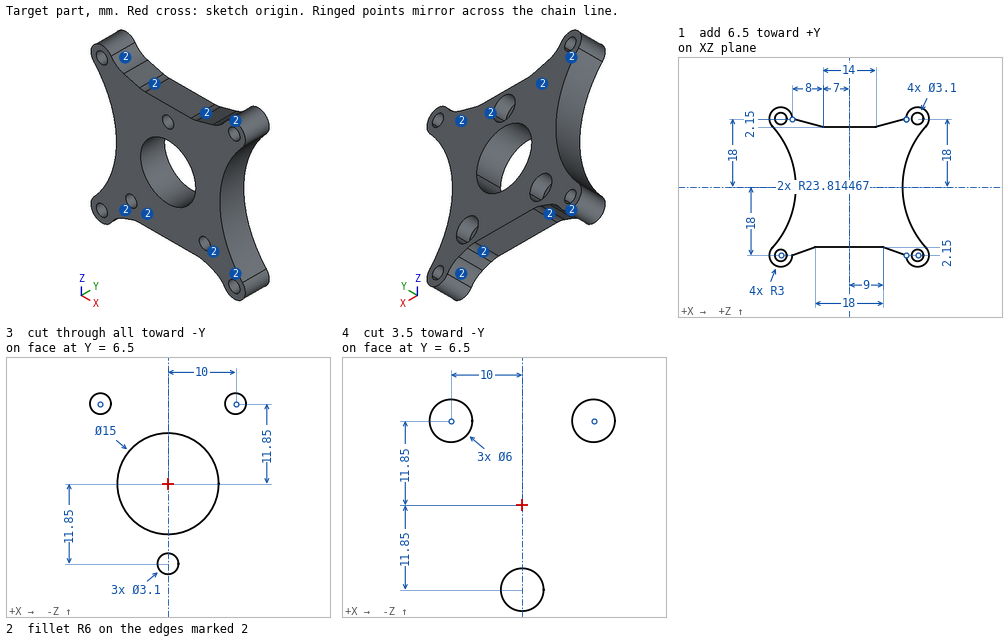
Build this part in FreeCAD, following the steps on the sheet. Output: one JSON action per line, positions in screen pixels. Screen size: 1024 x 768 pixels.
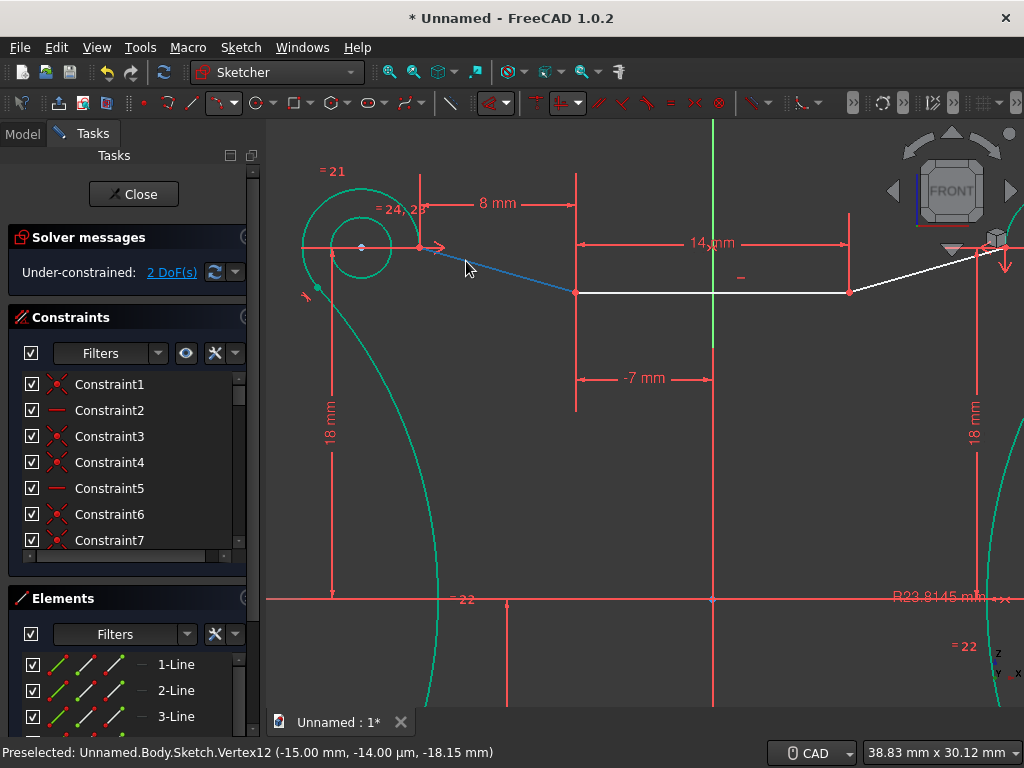
{"action": "left_click", "coordinate": [467, 261]}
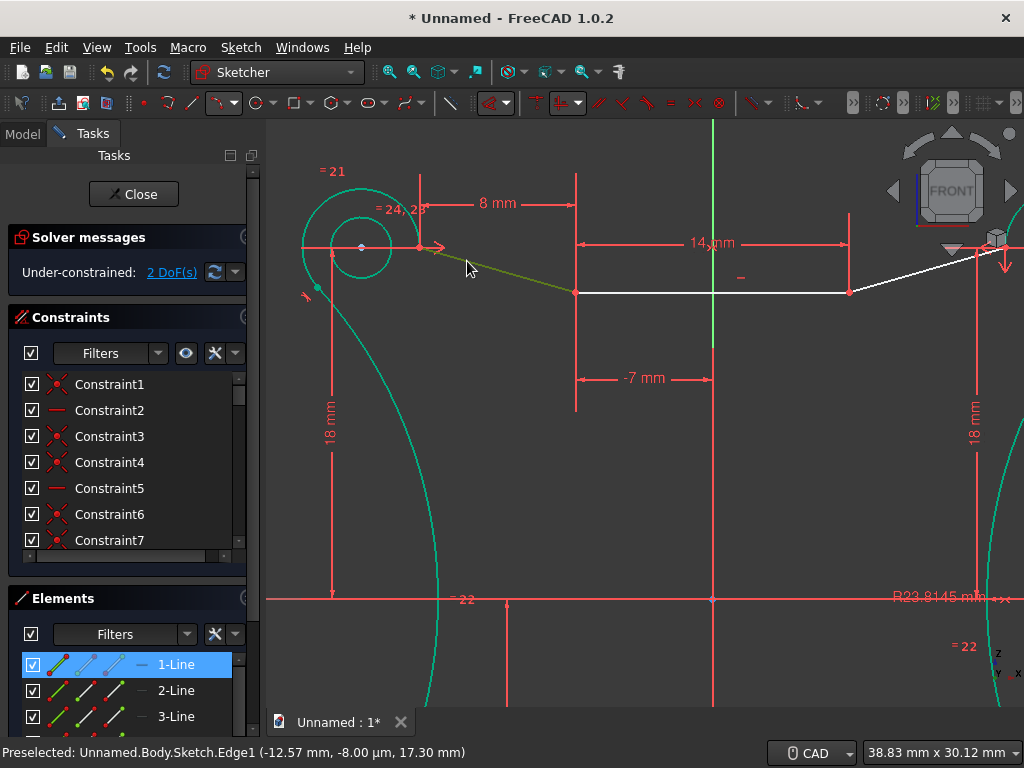
{"action": "key", "text": "i"}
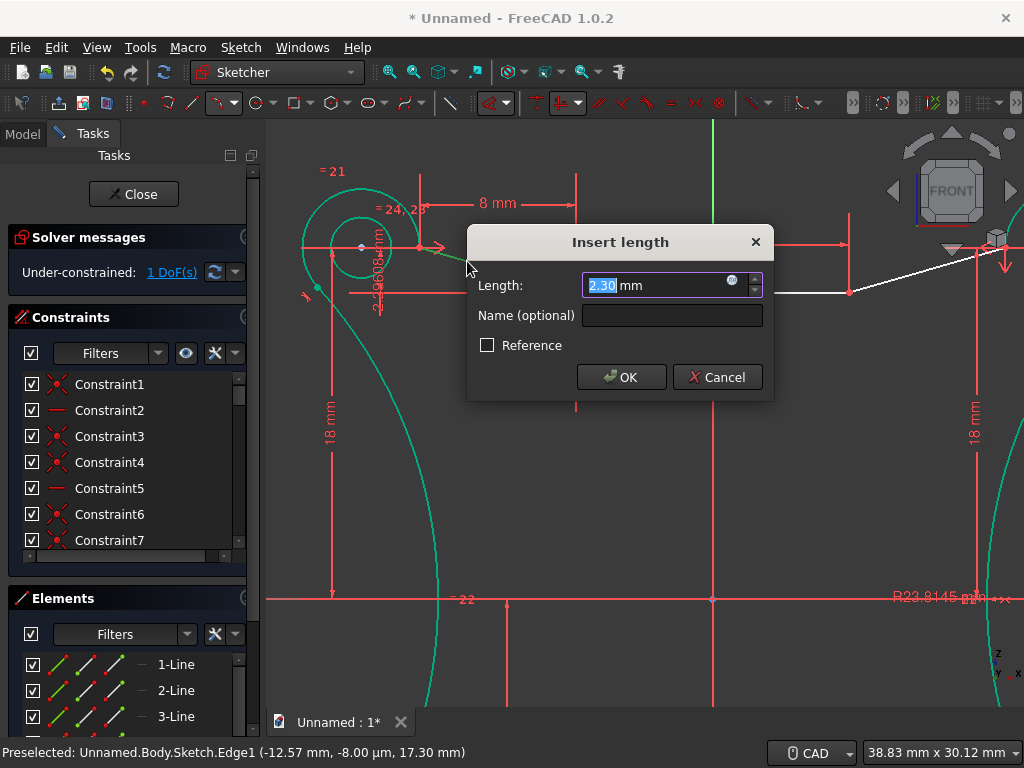
{"action": "type", "text": "2.15"}
{"action": "key", "text": "Return"}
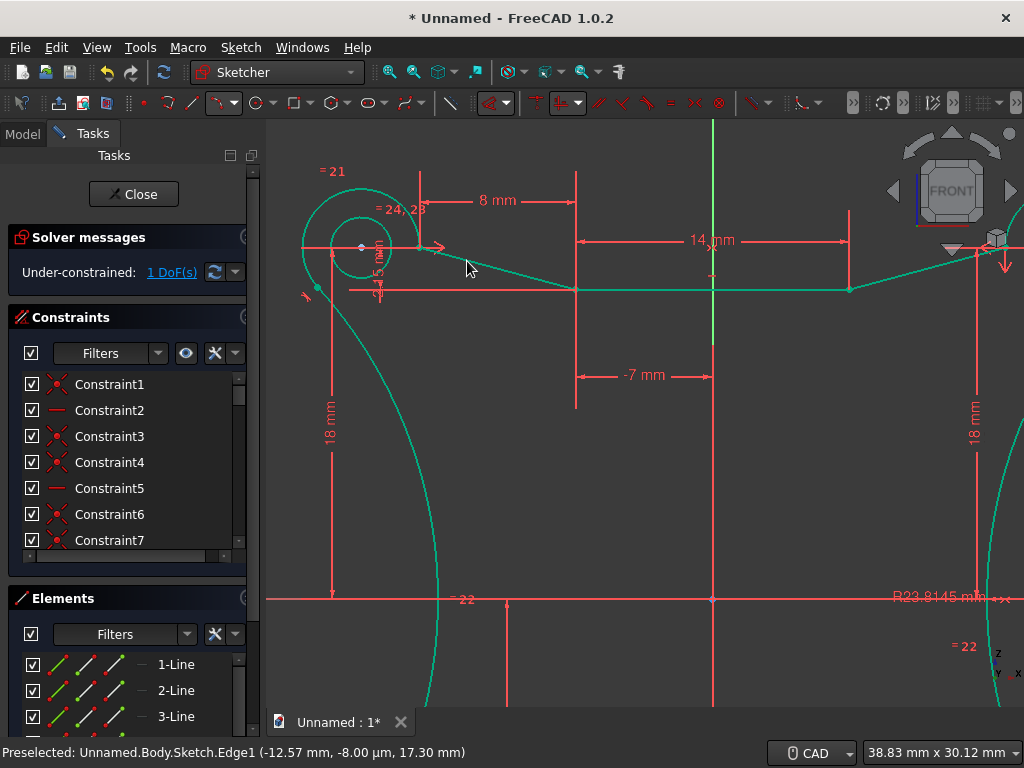
{"action": "scroll", "coordinate": [466, 261], "scroll_direction": "down", "scroll_amount": 4}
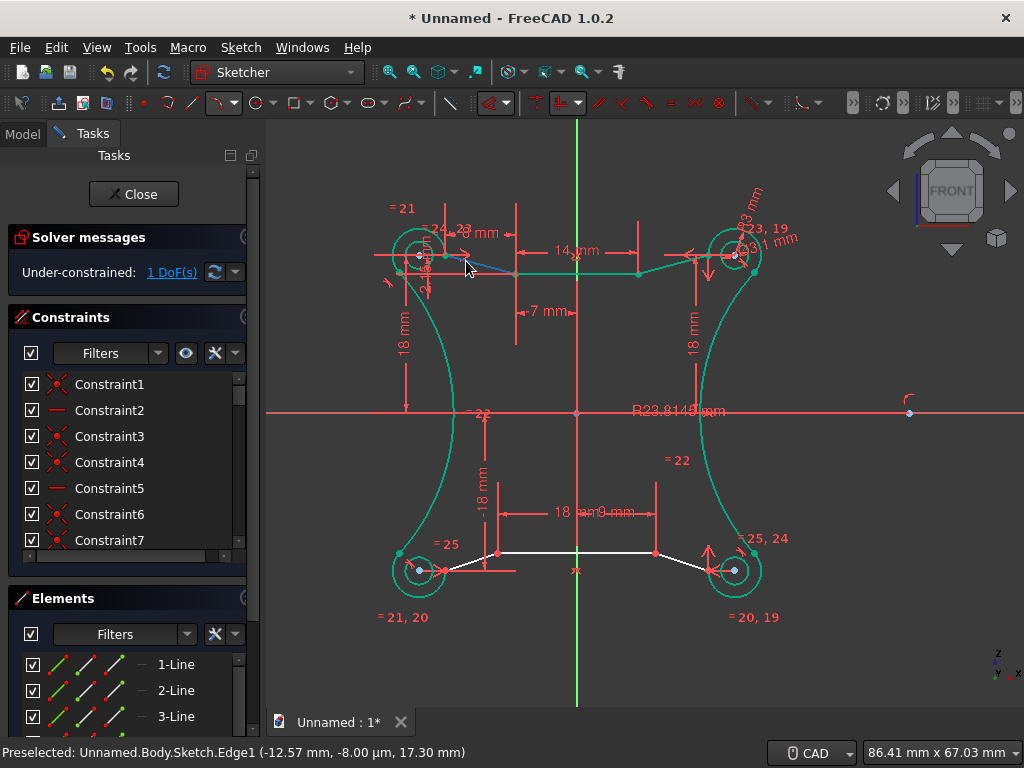
{"action": "scroll", "coordinate": [693, 566], "scroll_direction": "up", "scroll_amount": 4}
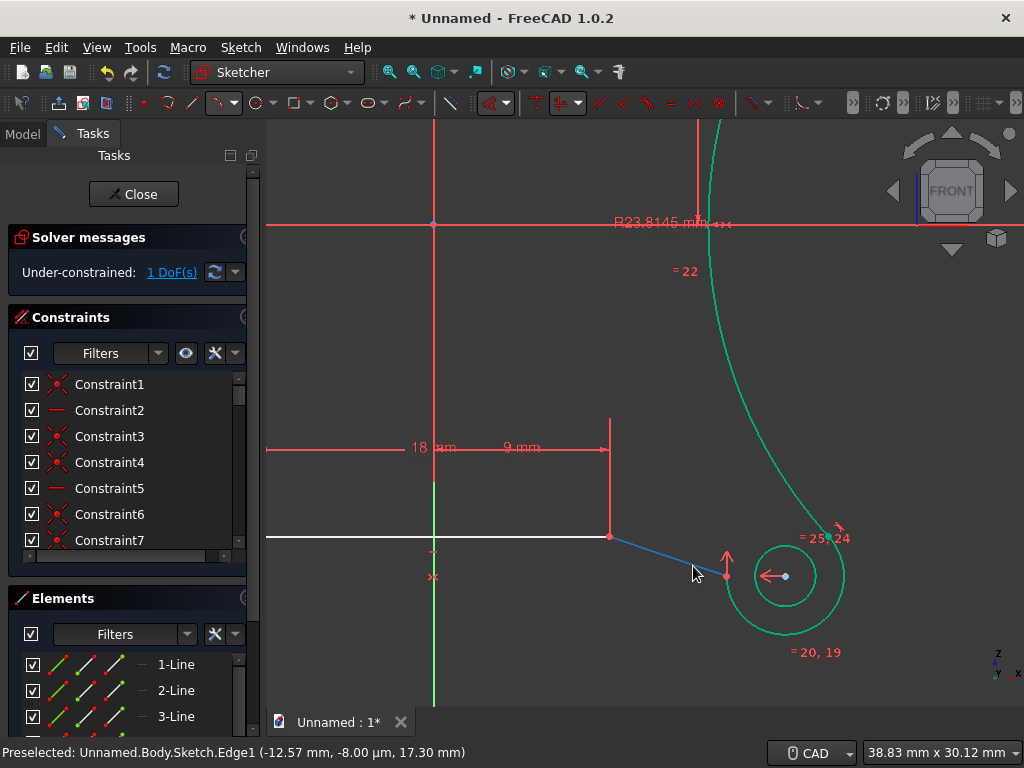
{"action": "left_click", "coordinate": [692, 564]}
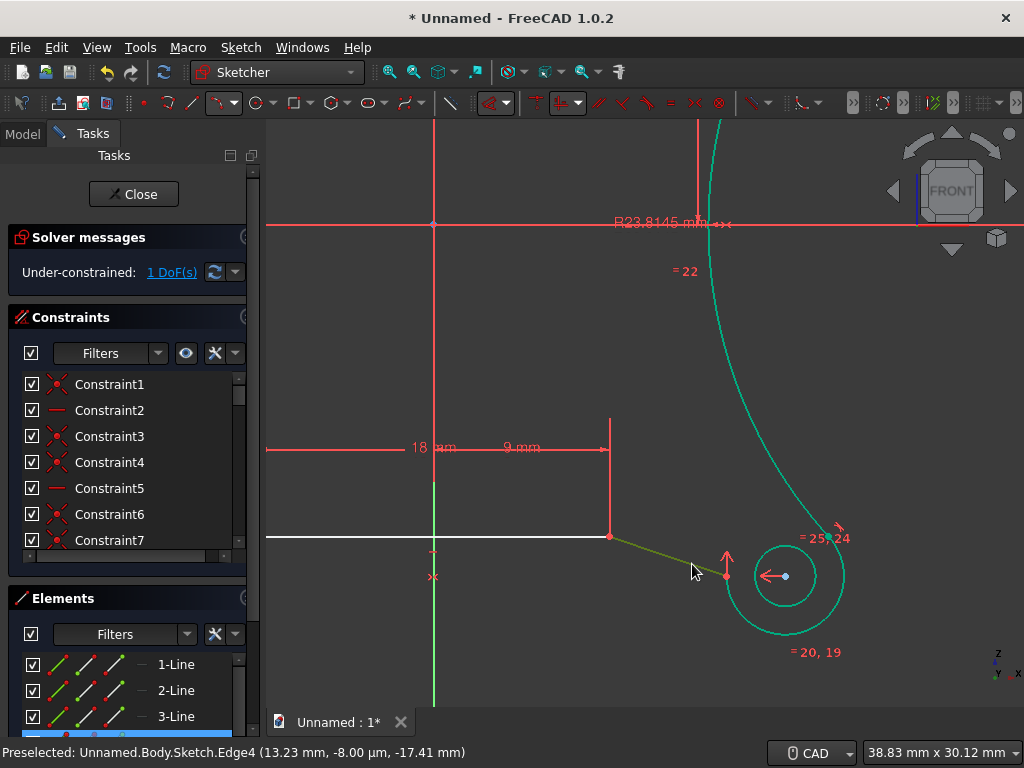
{"action": "left_click", "coordinate": [508, 104]}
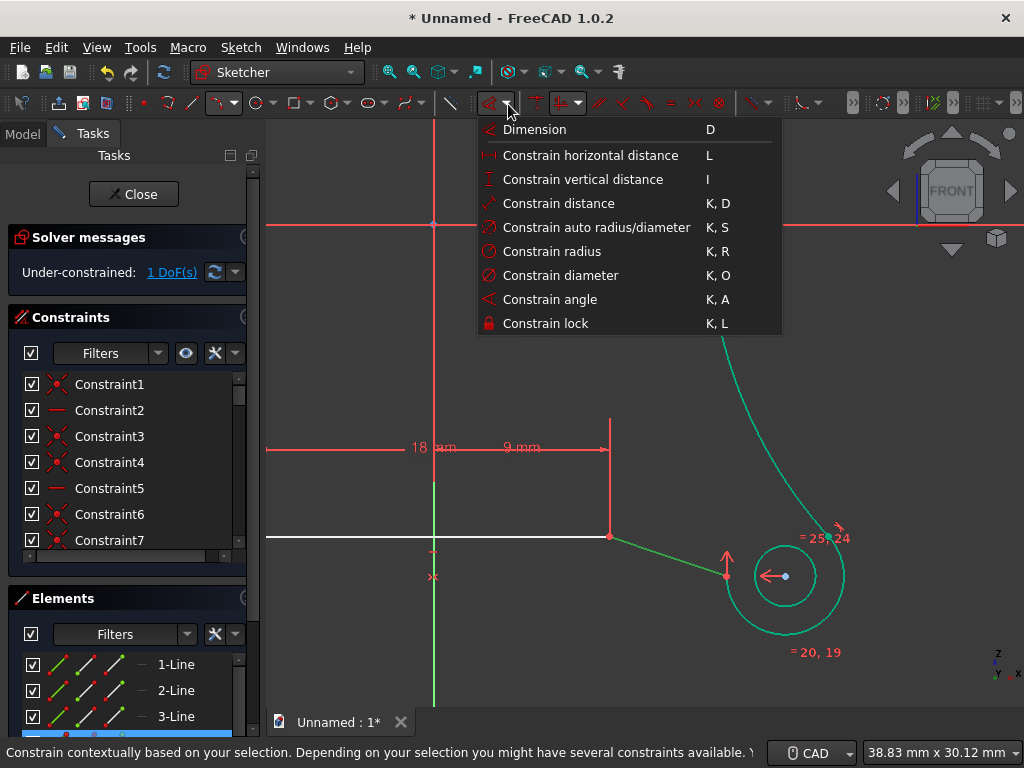
{"action": "left_click", "coordinate": [630, 179]}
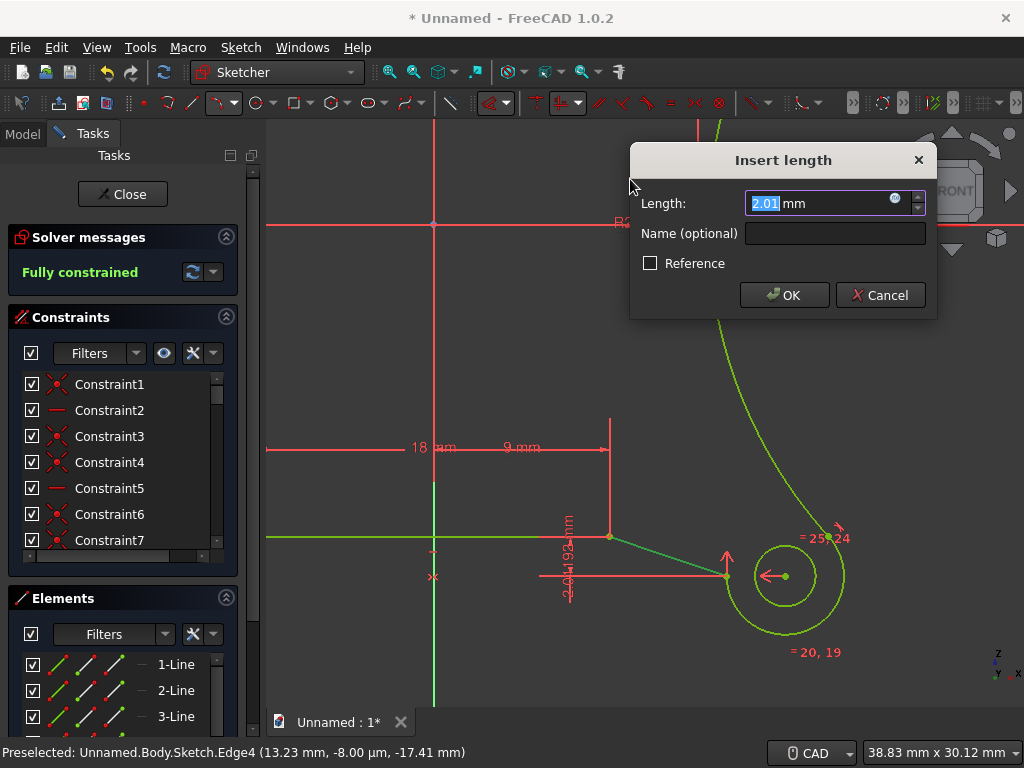
{"action": "type", "text": "2.15"}
{"action": "key", "text": "Return"}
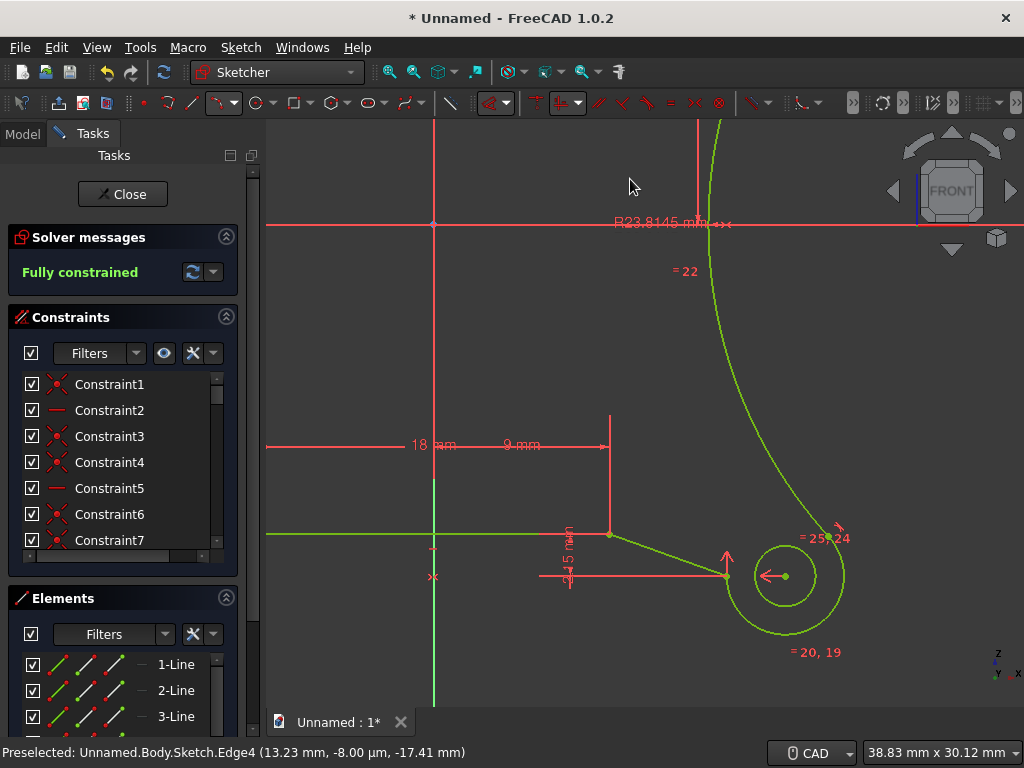
{"action": "left_click", "coordinate": [123, 194]}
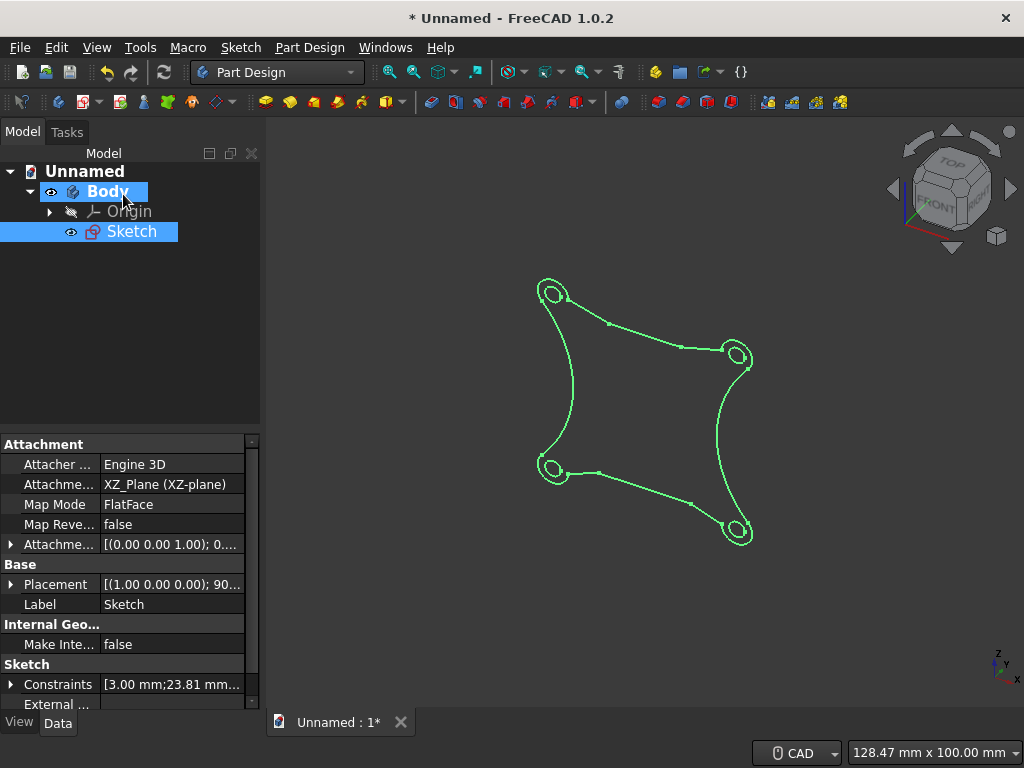
{"action": "left_click", "coordinate": [266, 102]}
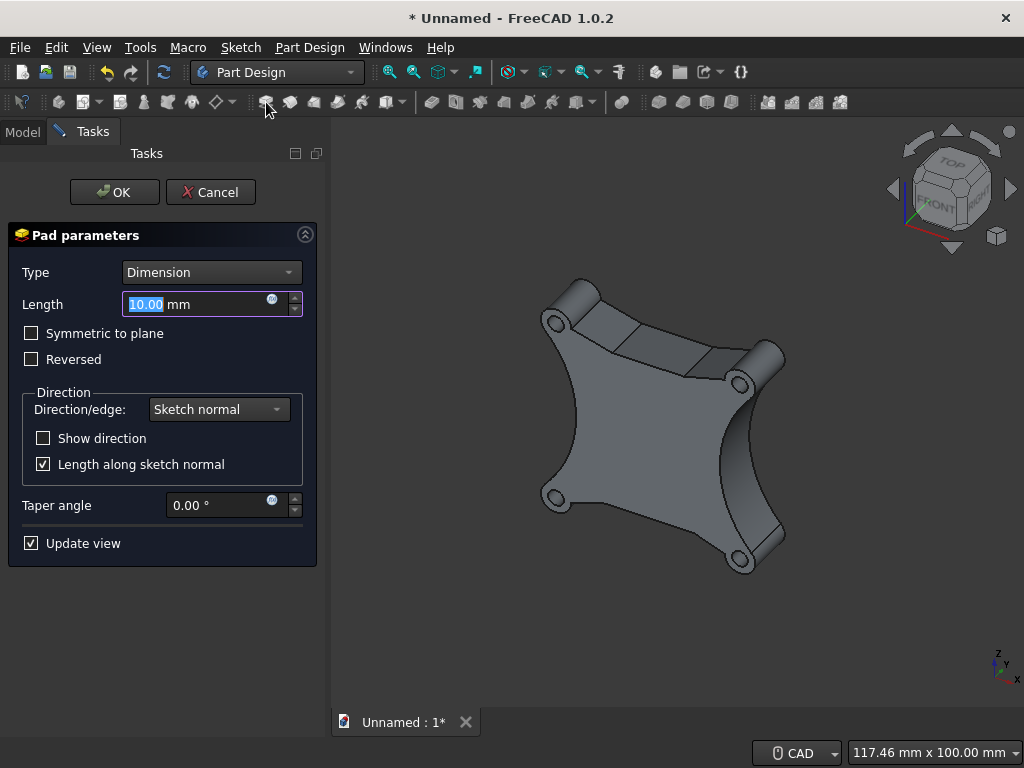
{"action": "type", "text": "6.5"}
{"action": "key", "text": "Tab"}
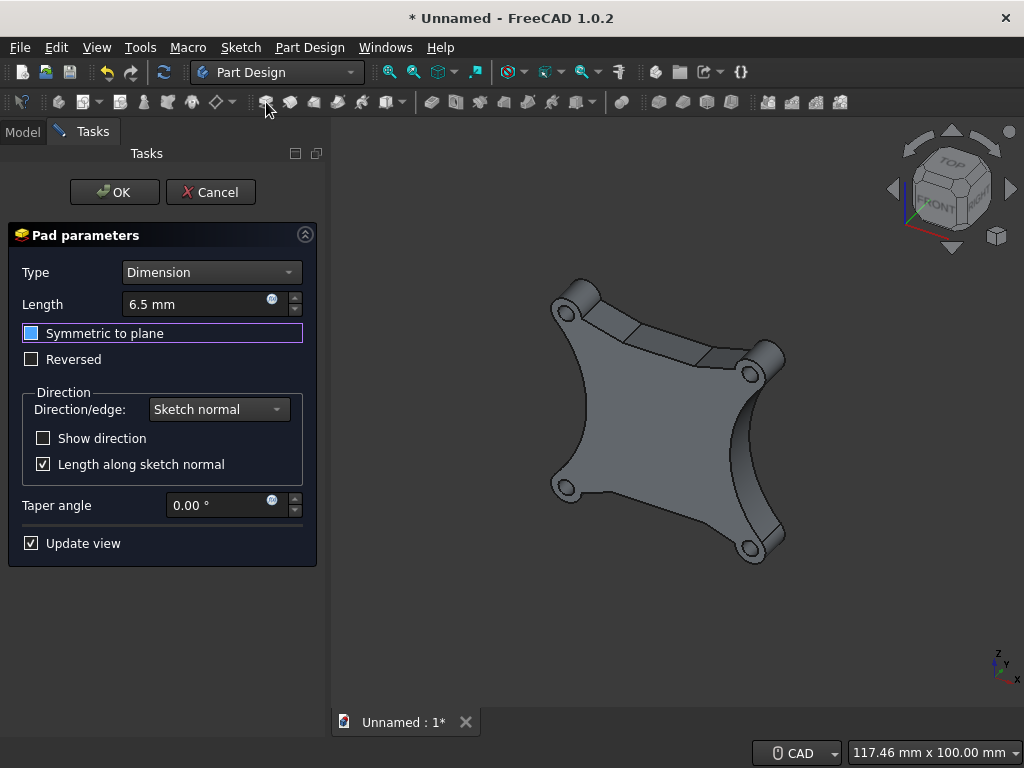
{"action": "left_click", "coordinate": [30, 359]}